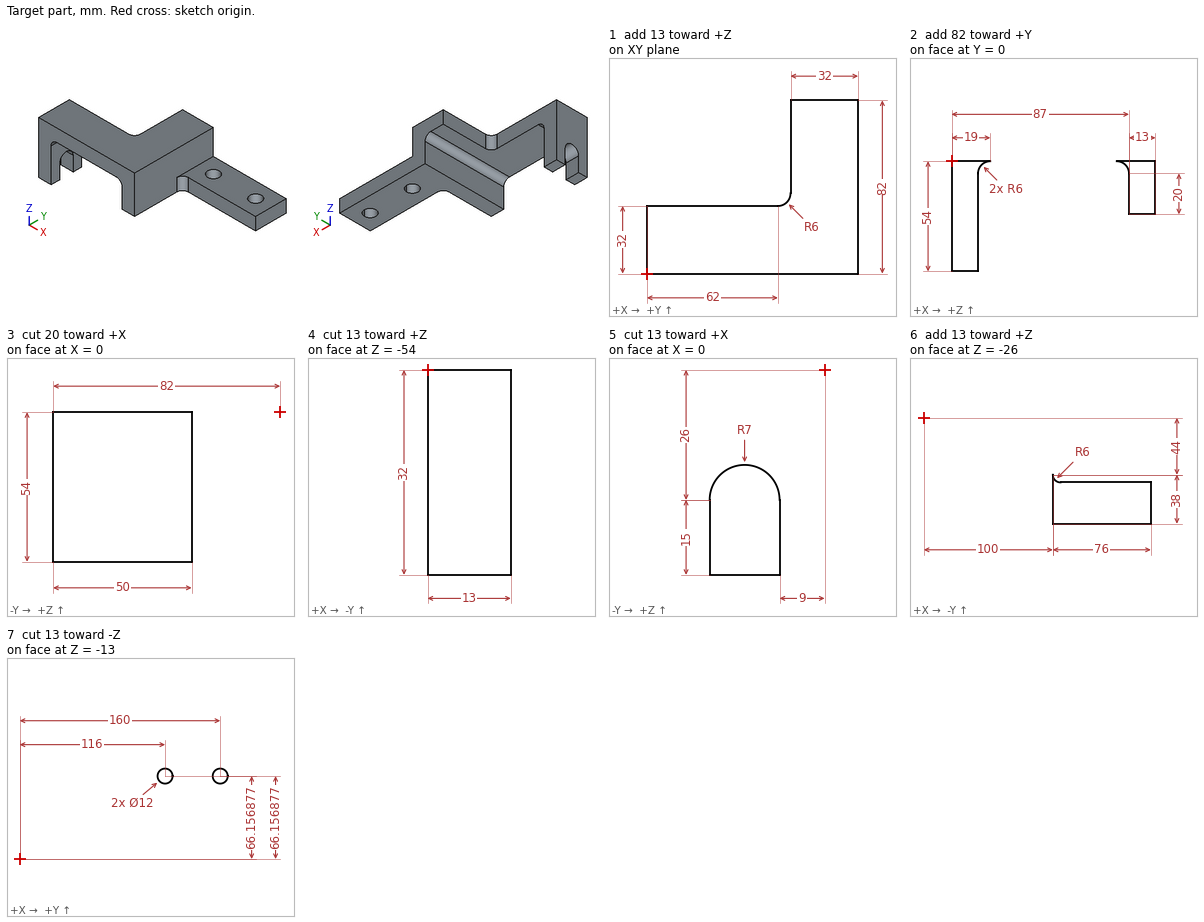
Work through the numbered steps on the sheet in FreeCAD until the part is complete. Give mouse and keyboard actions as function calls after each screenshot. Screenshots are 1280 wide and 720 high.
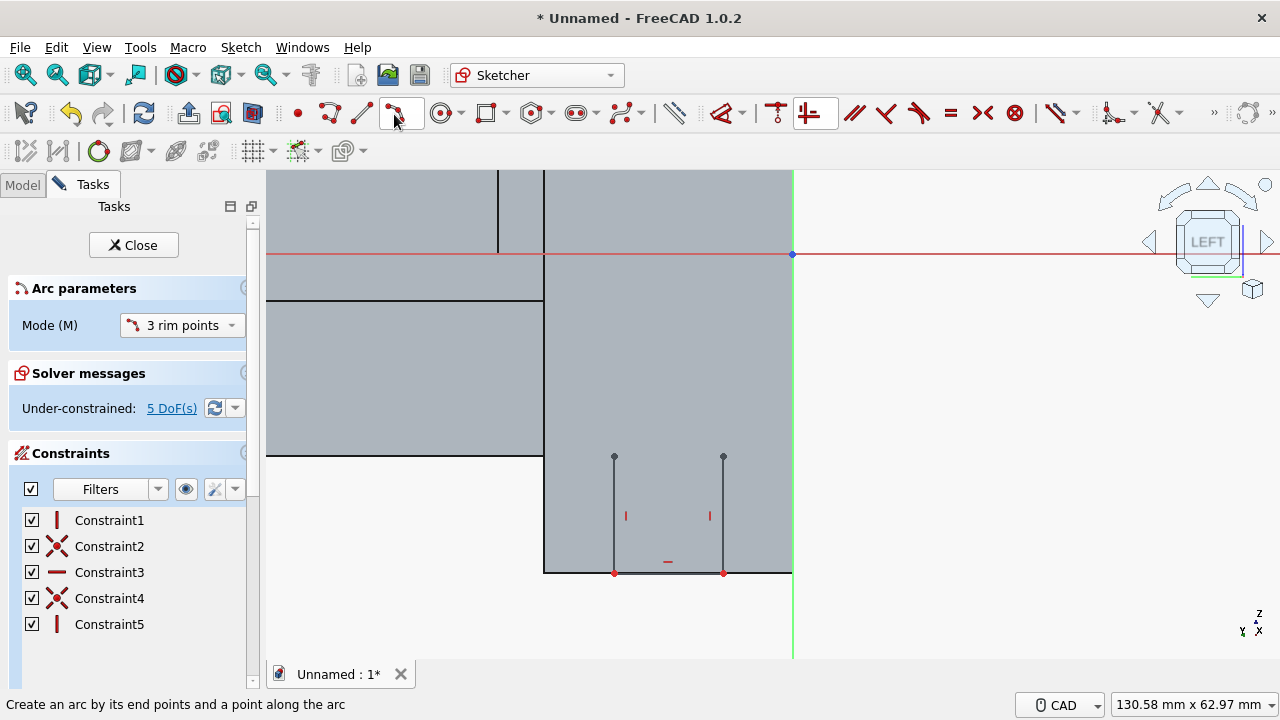
click(723, 457)
click(614, 457)
click(668, 402)
key(Escape)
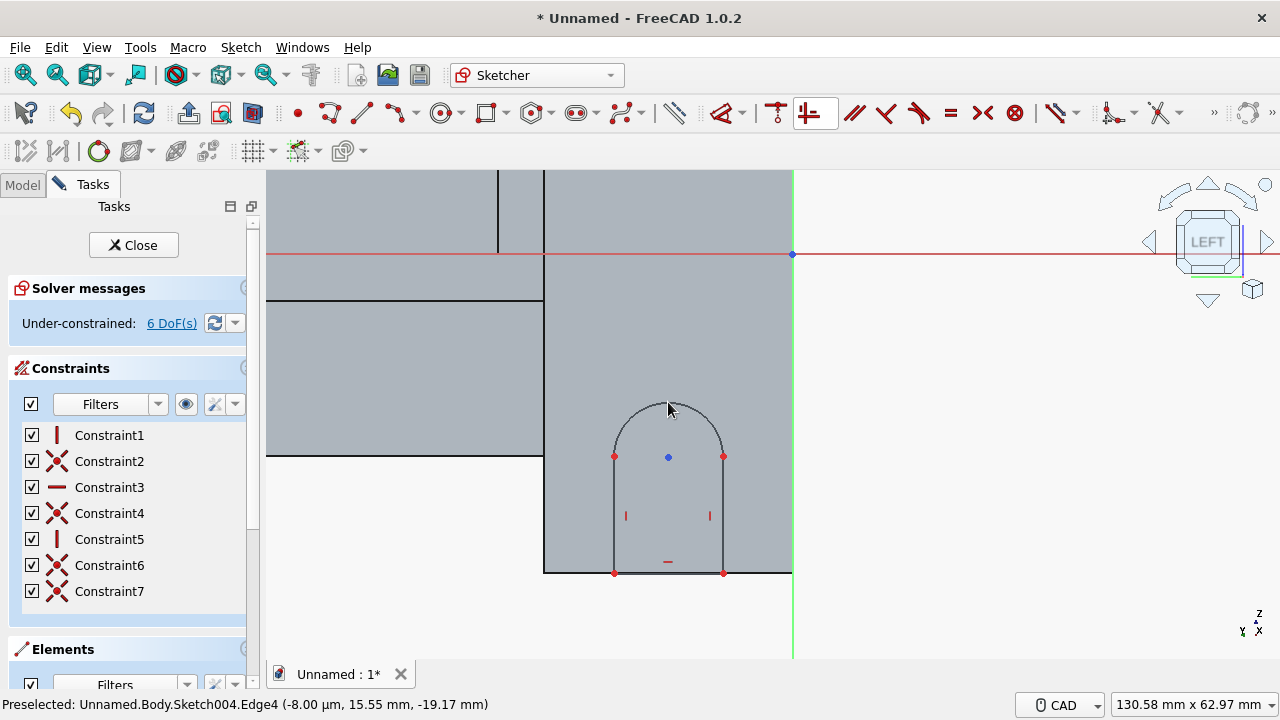
click(614, 492)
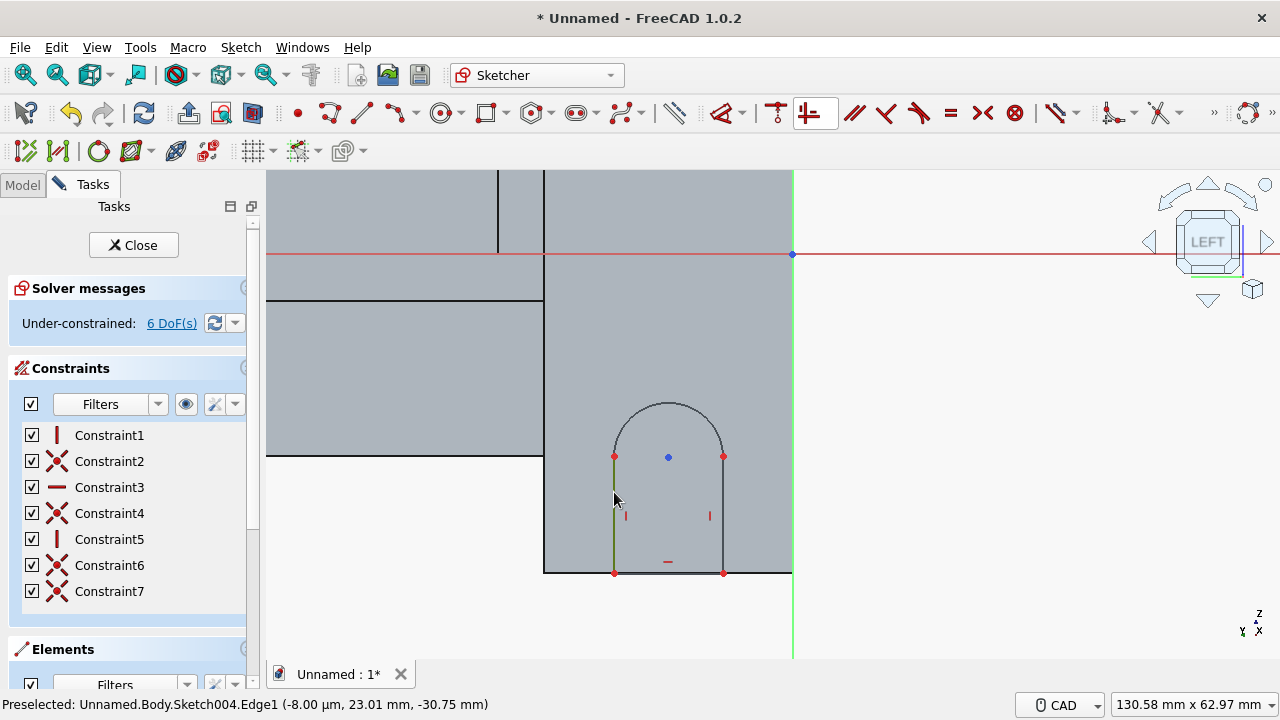
click(700, 413)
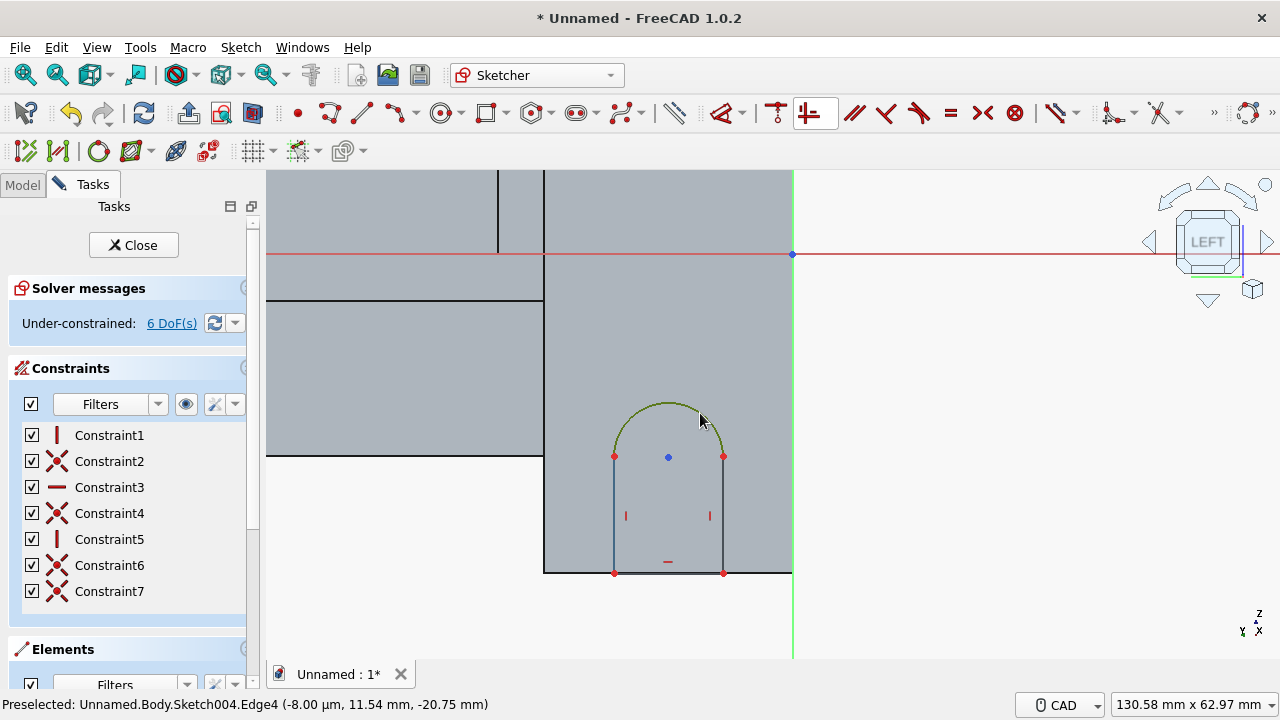
click(920, 114)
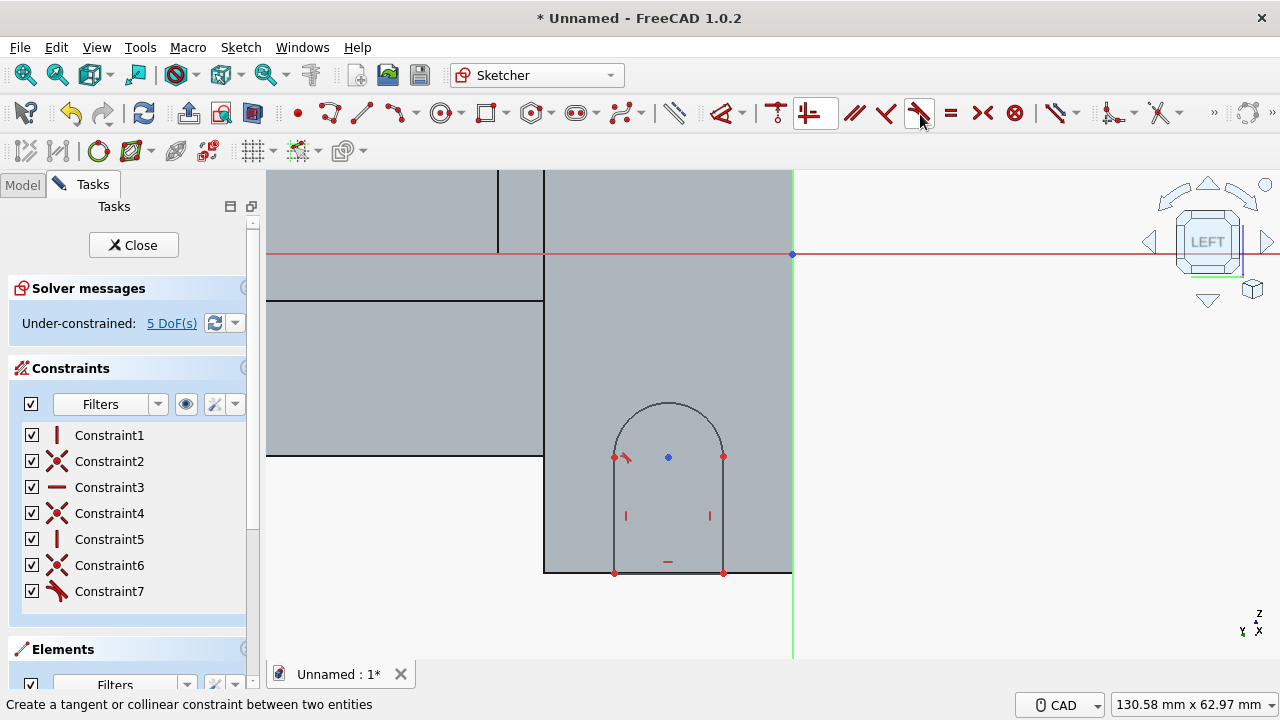
click(723, 539)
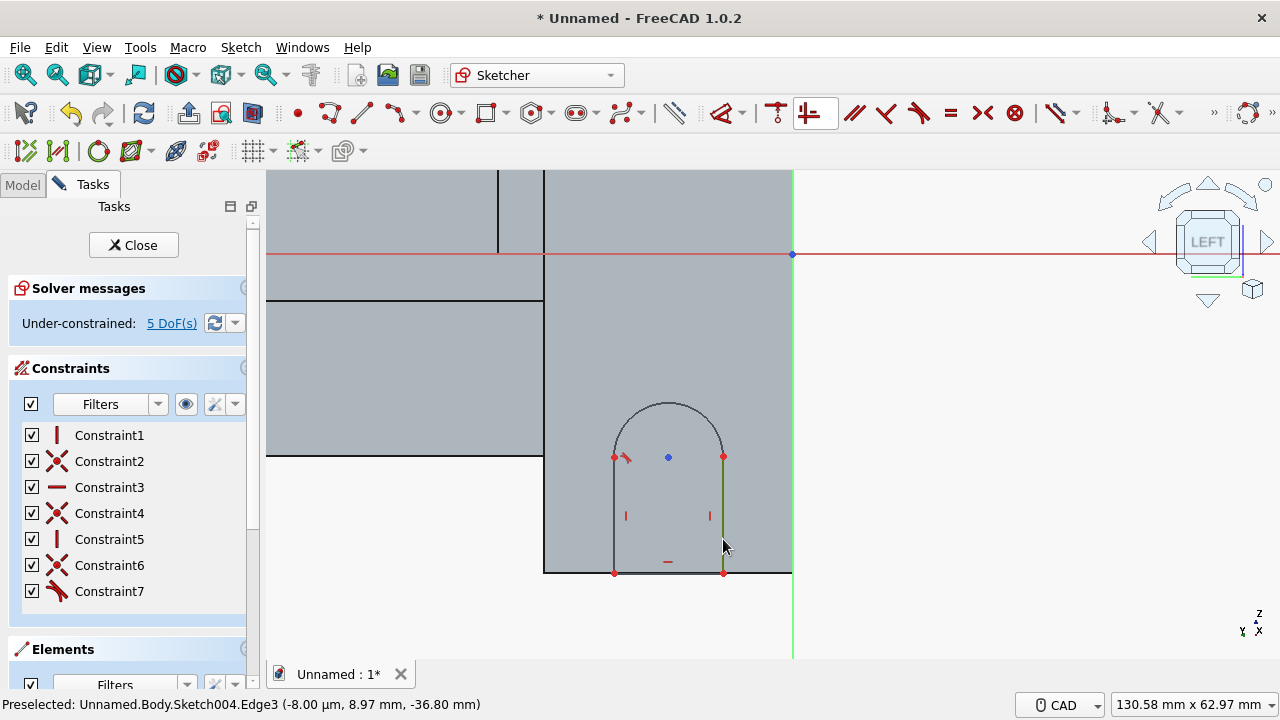
click(700, 413)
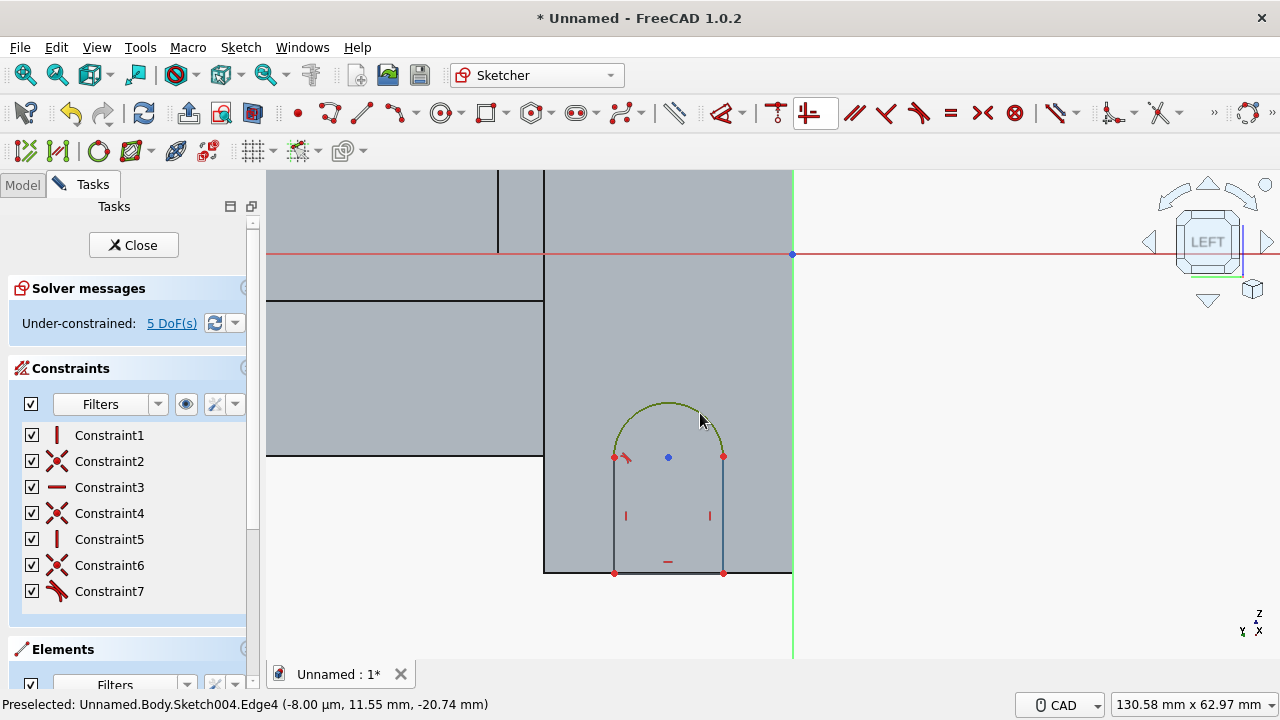
click(920, 114)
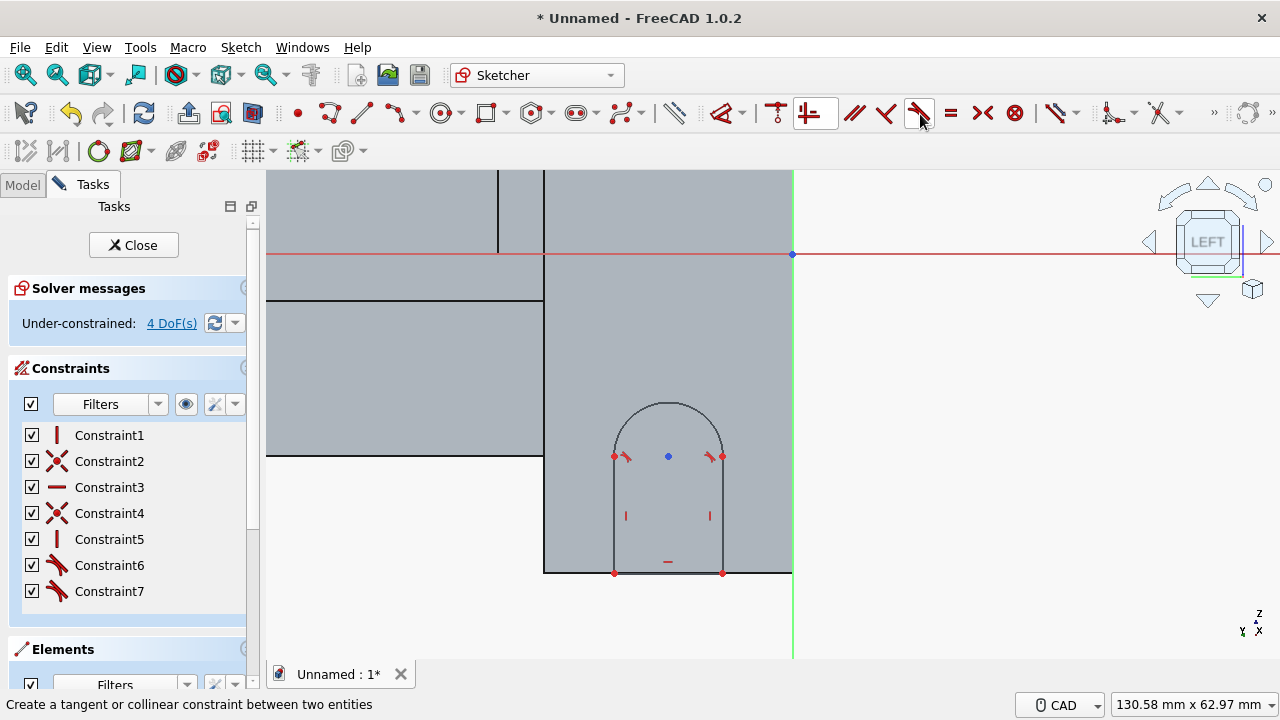
click(722, 114)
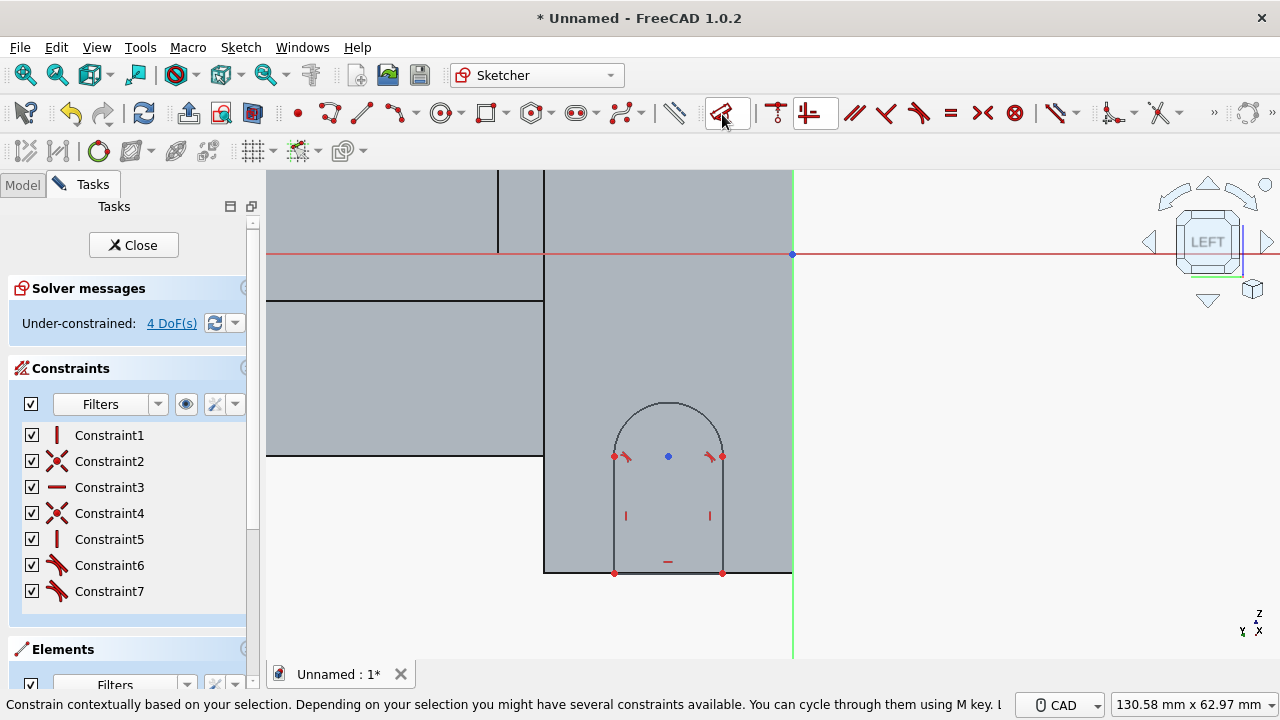
click(701, 413)
click(720, 387)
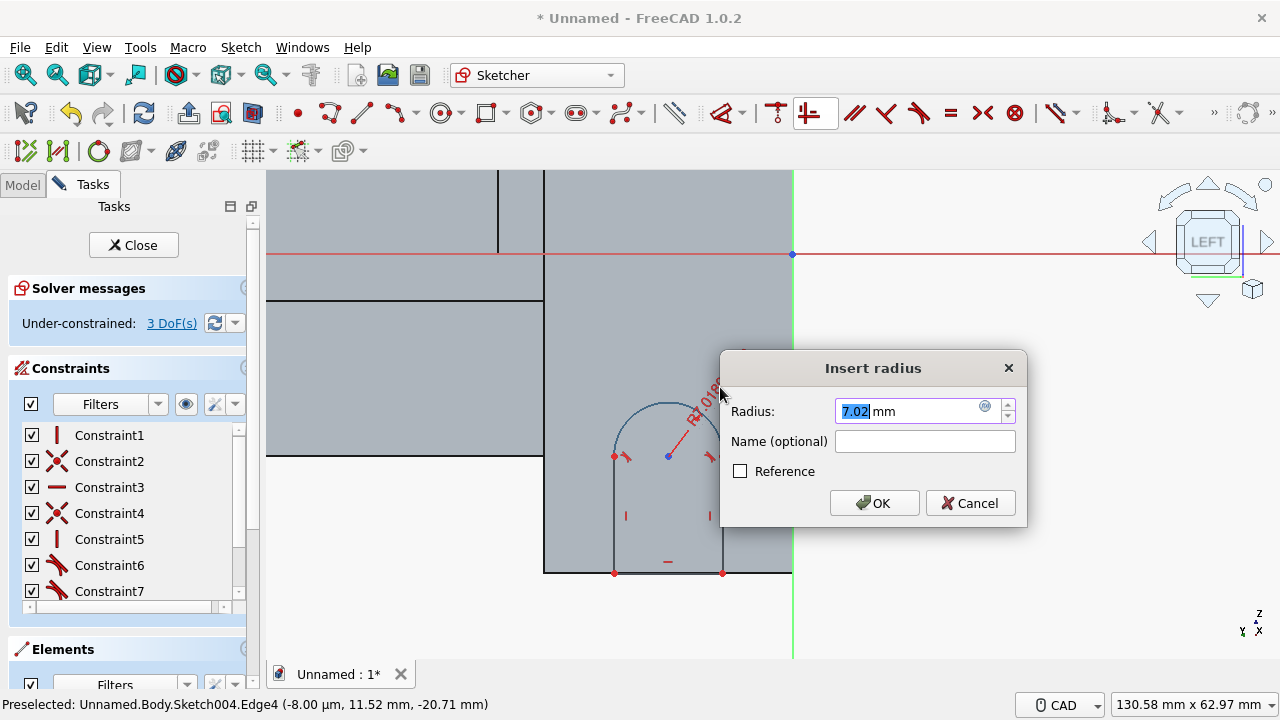
text(7)
key(Return)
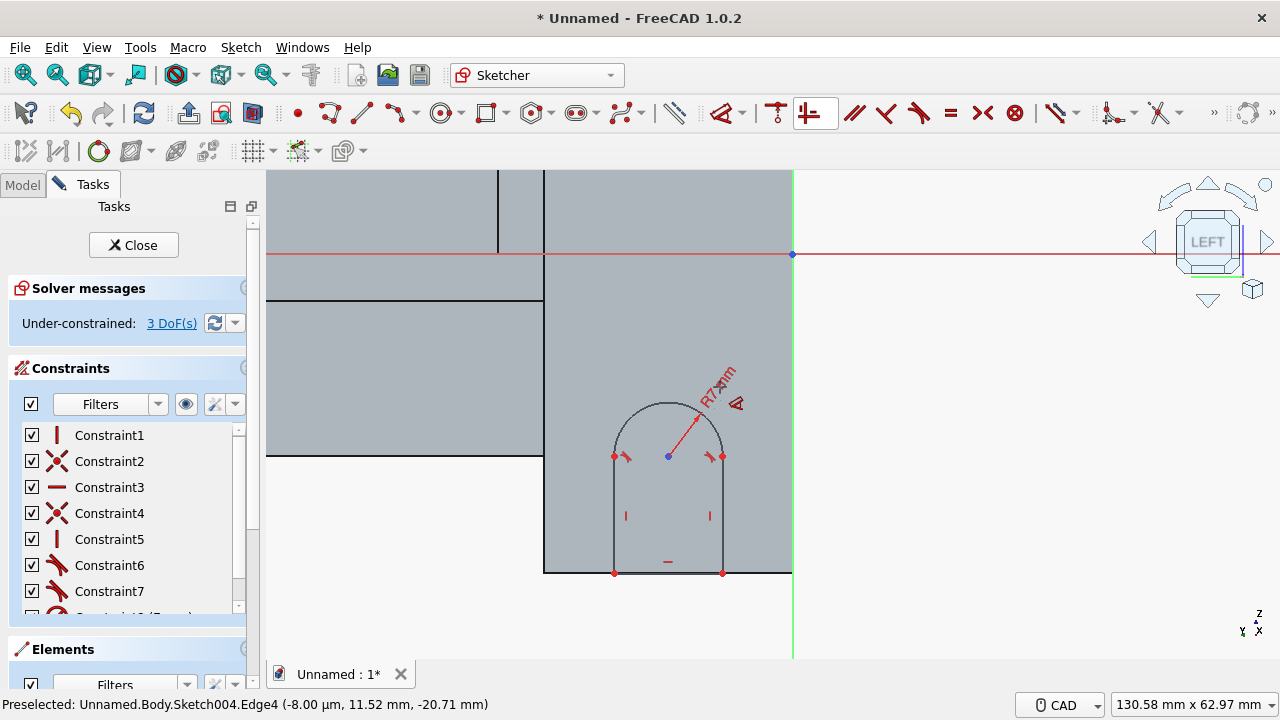
click(614, 492)
click(580, 515)